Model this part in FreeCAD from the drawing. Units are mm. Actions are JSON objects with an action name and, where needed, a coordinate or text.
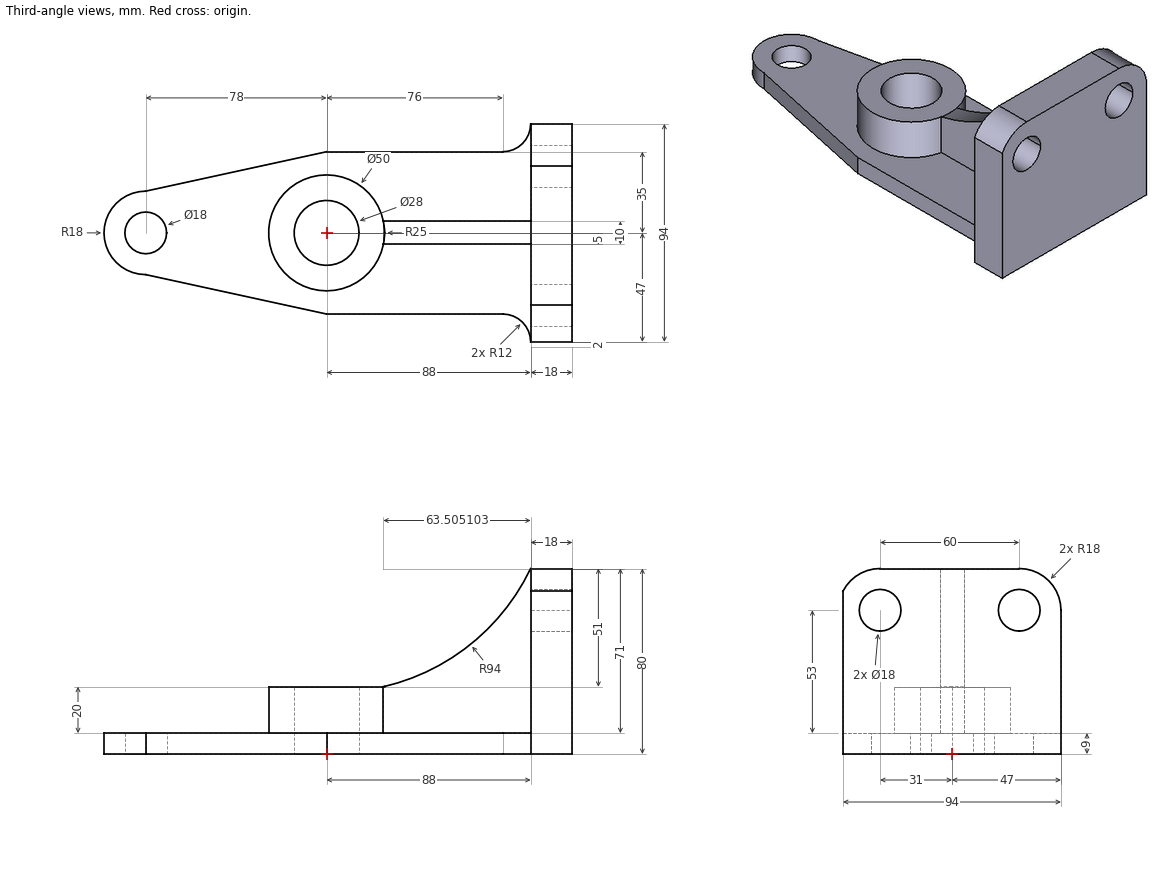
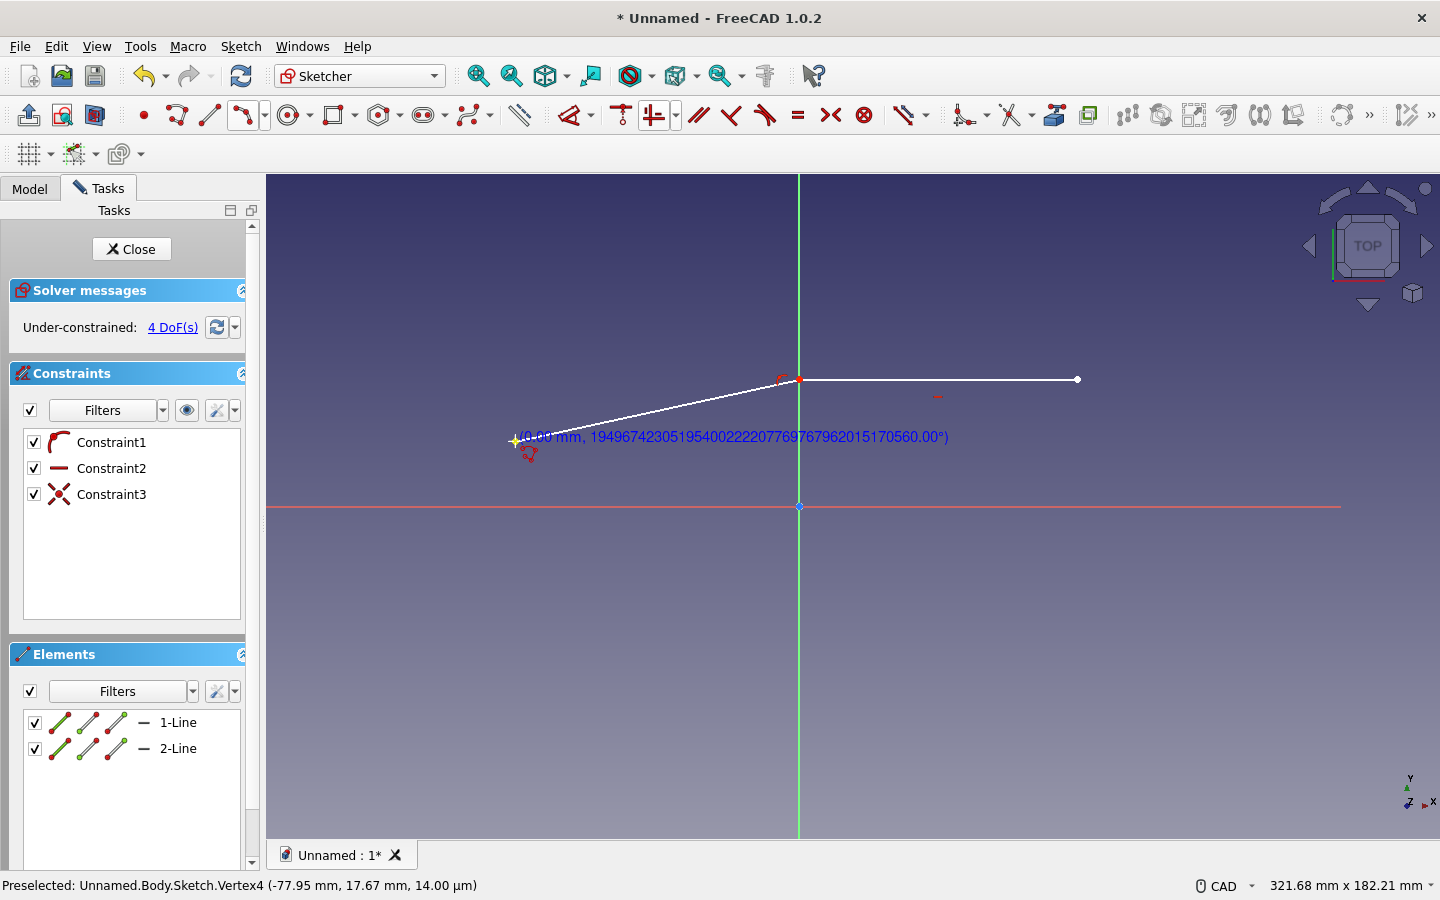
{"action": "left_click", "coordinate": [515, 572]}
{"action": "left_click", "coordinate": [799, 634]}
{"action": "left_click", "coordinate": [1077, 634]}
{"action": "right_click", "coordinate": [1077, 634]}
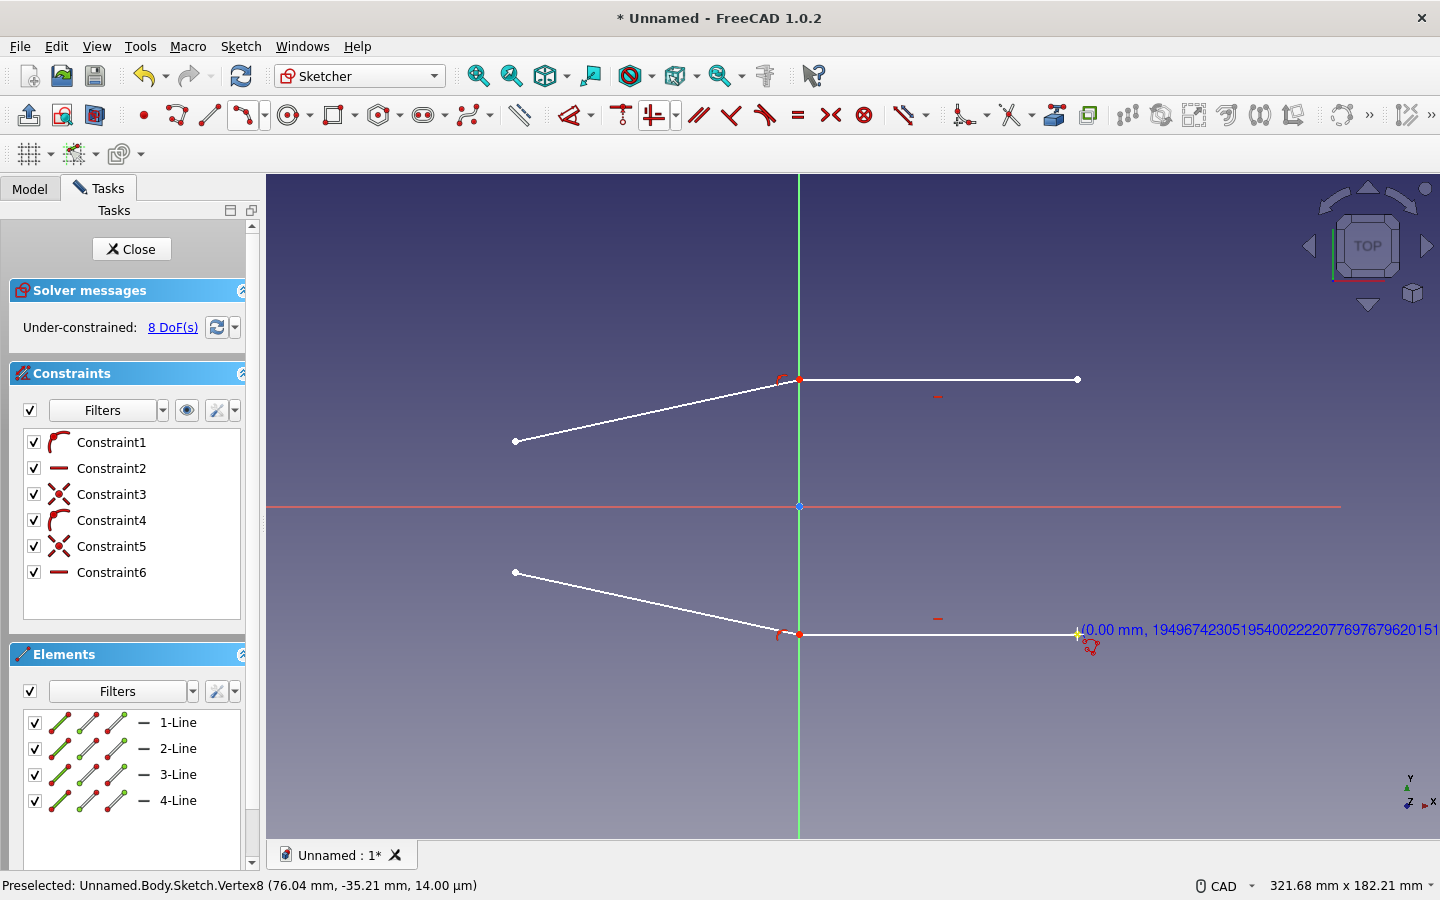
{"action": "left_click", "coordinate": [210, 116]}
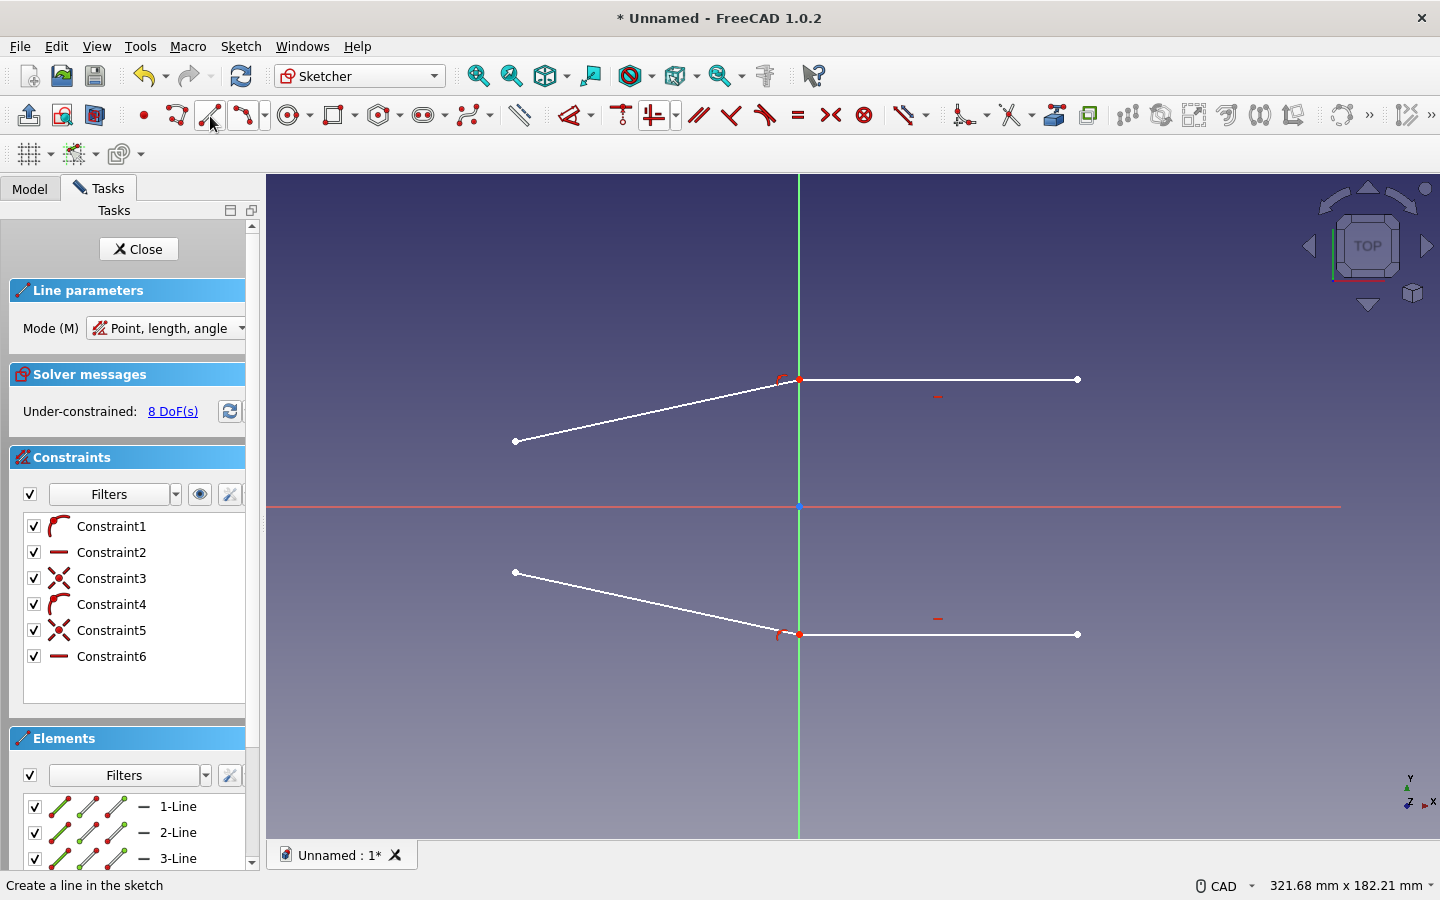
{"action": "left_click", "coordinate": [1121, 678]}
{"action": "left_click", "coordinate": [1121, 335]}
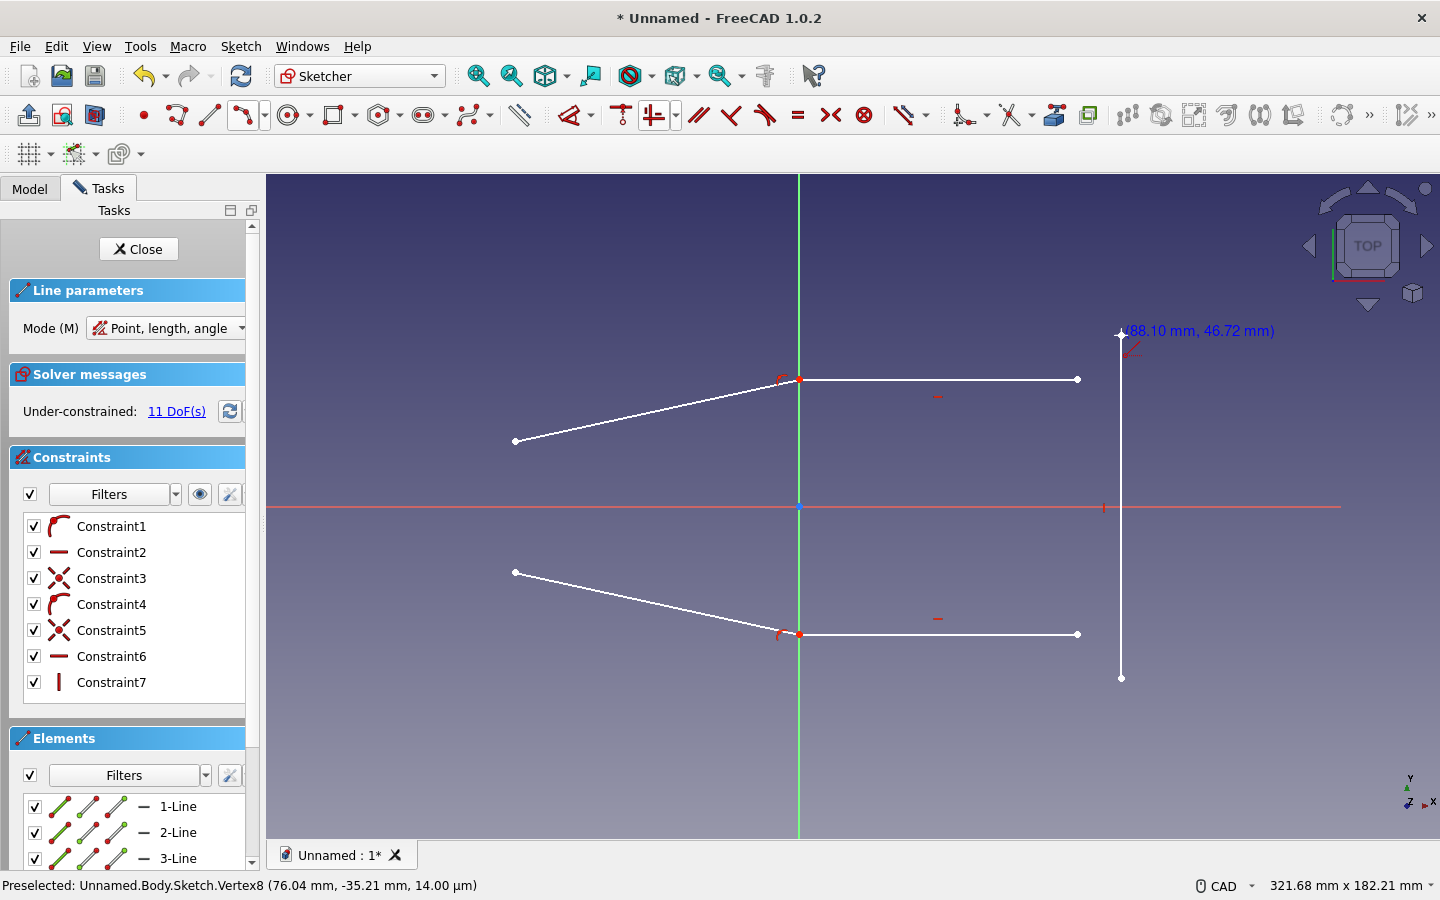
{"action": "left_click", "coordinate": [242, 116]}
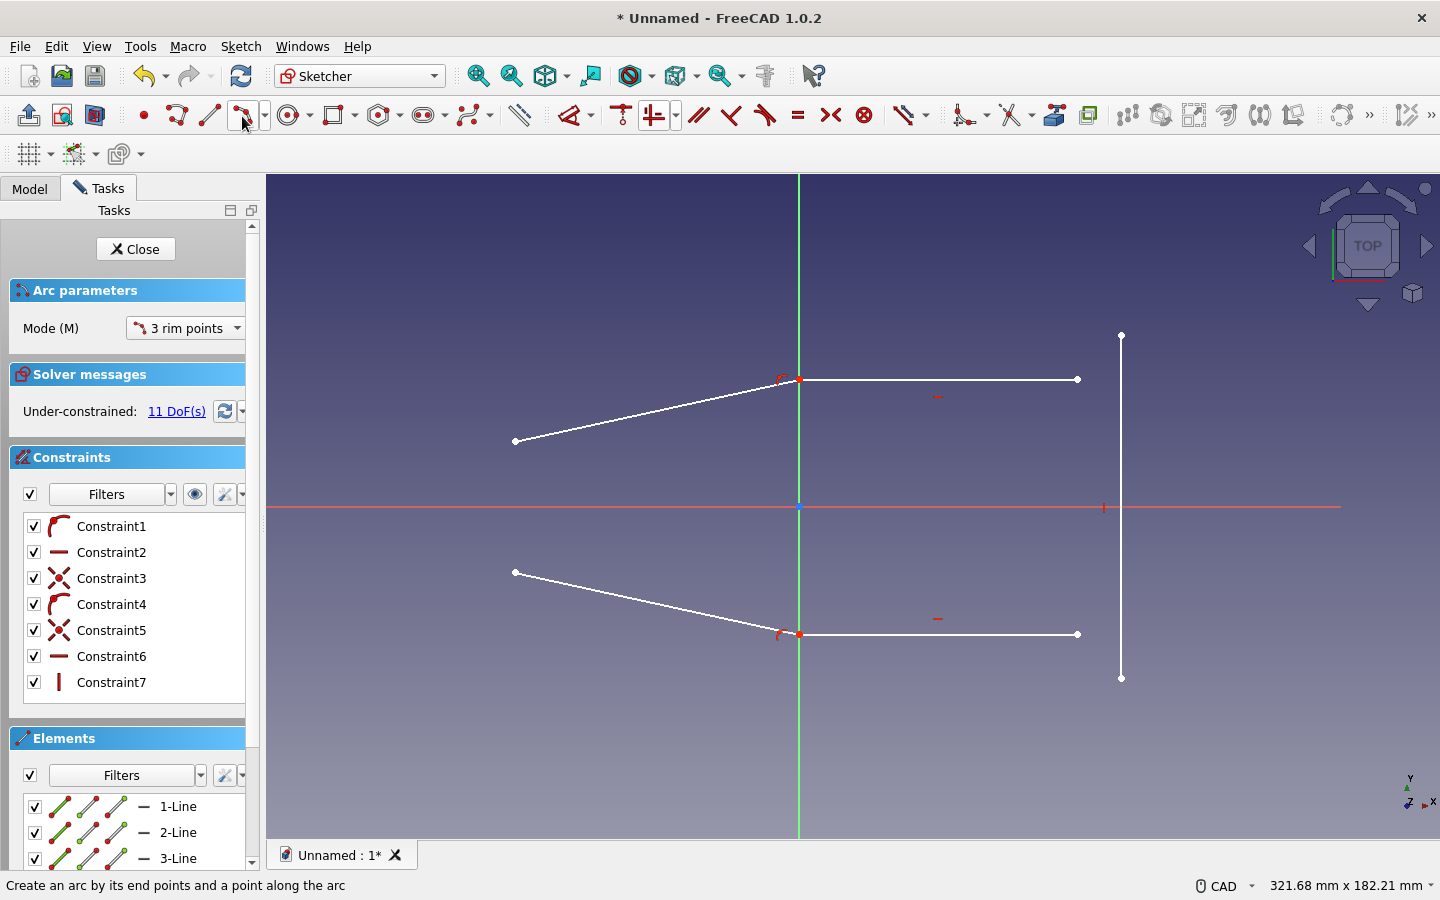
{"action": "left_click", "coordinate": [515, 442]}
{"action": "left_click", "coordinate": [515, 573]}
{"action": "left_click", "coordinate": [452, 486]}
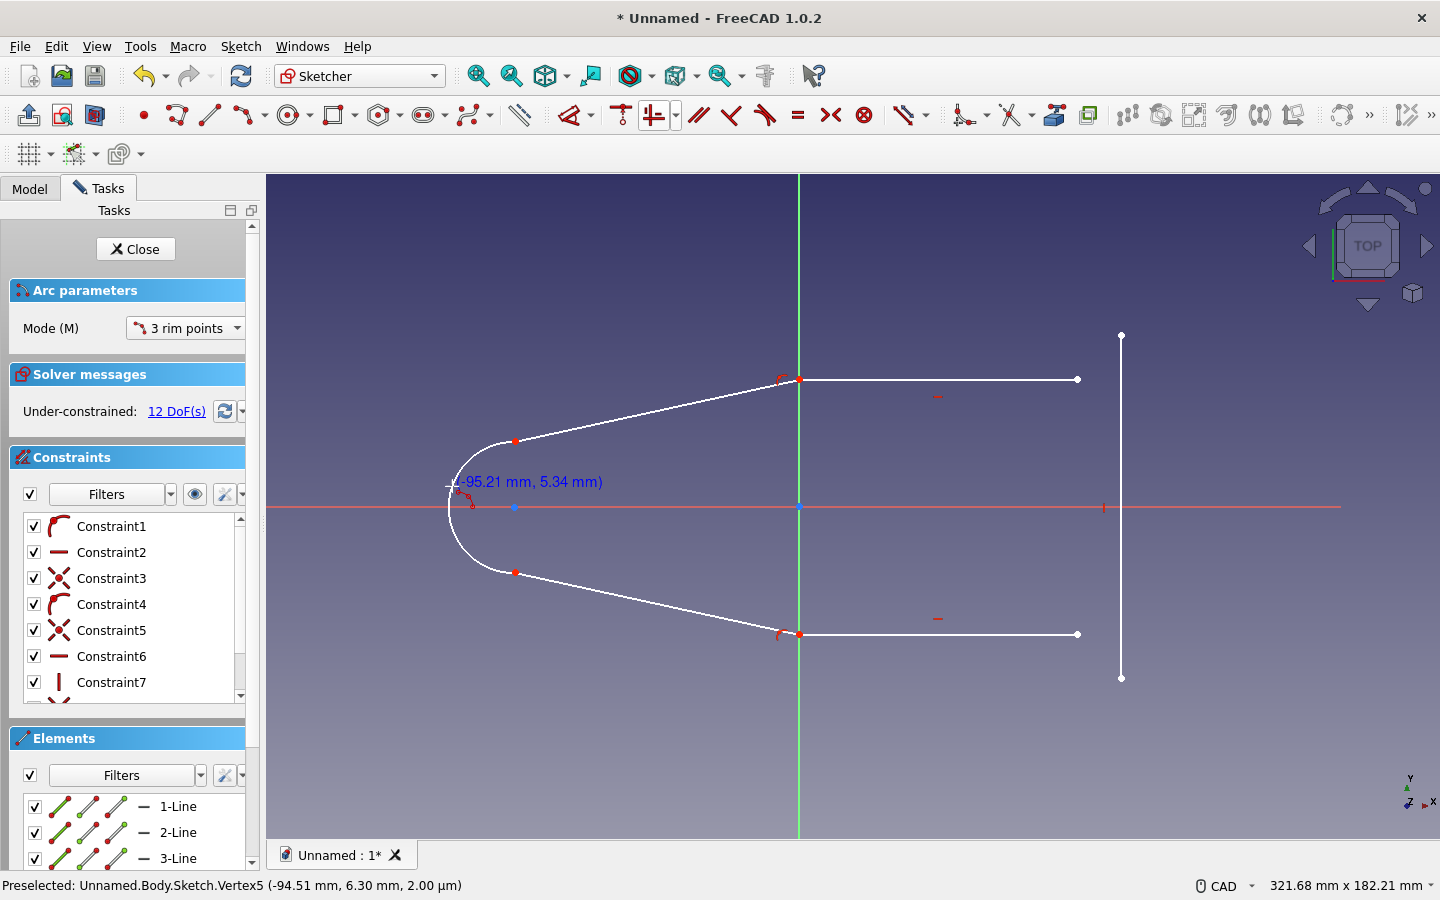
{"action": "left_click", "coordinate": [1077, 635]}
{"action": "left_click", "coordinate": [1121, 679]}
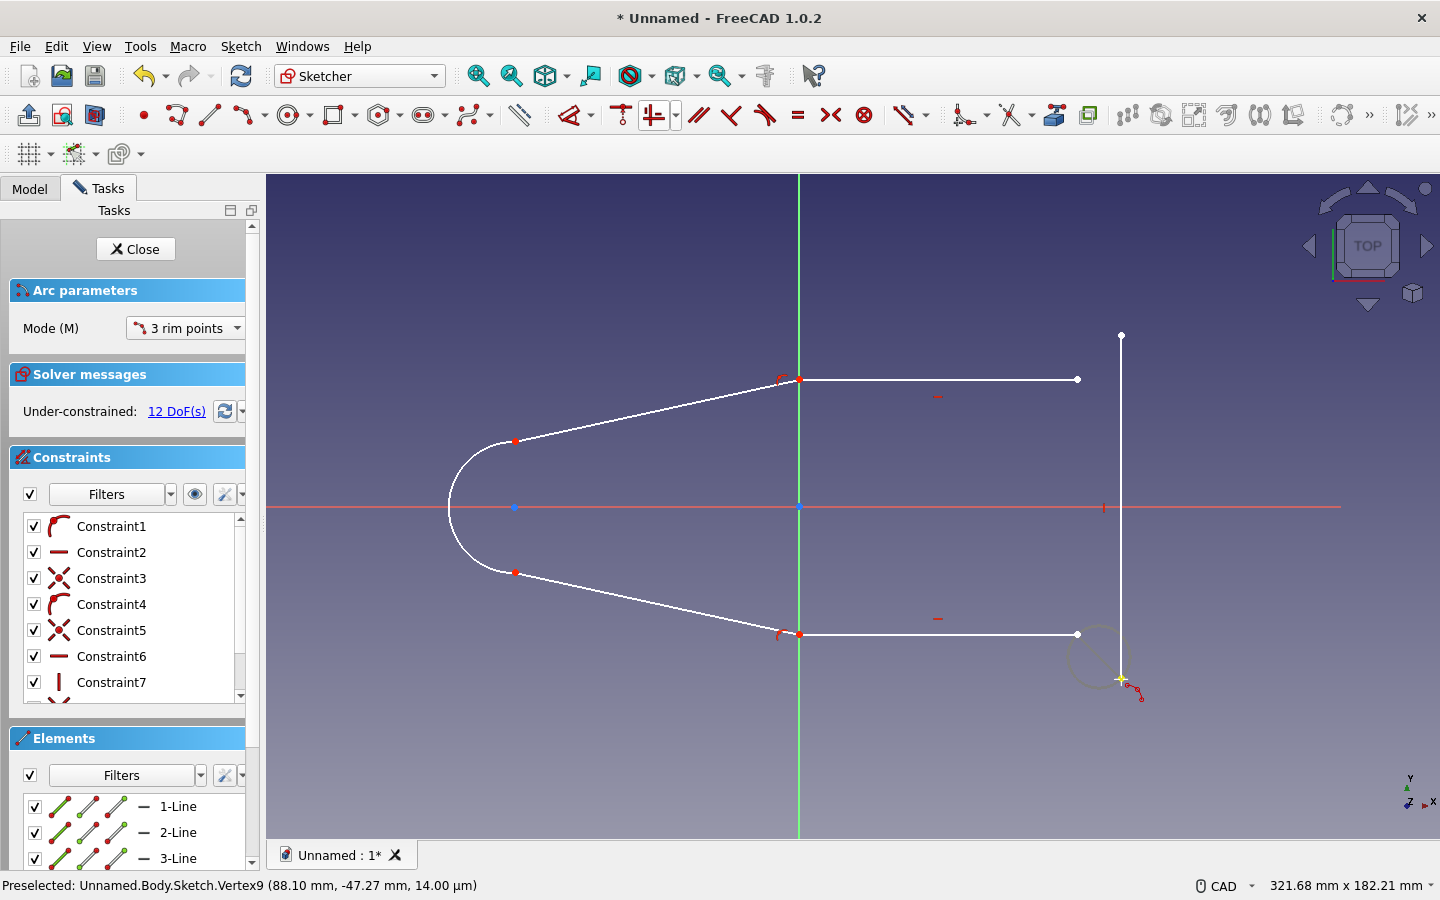
{"action": "scroll", "coordinate": [1108, 647], "scroll_direction": "up", "scroll_amount": 2}